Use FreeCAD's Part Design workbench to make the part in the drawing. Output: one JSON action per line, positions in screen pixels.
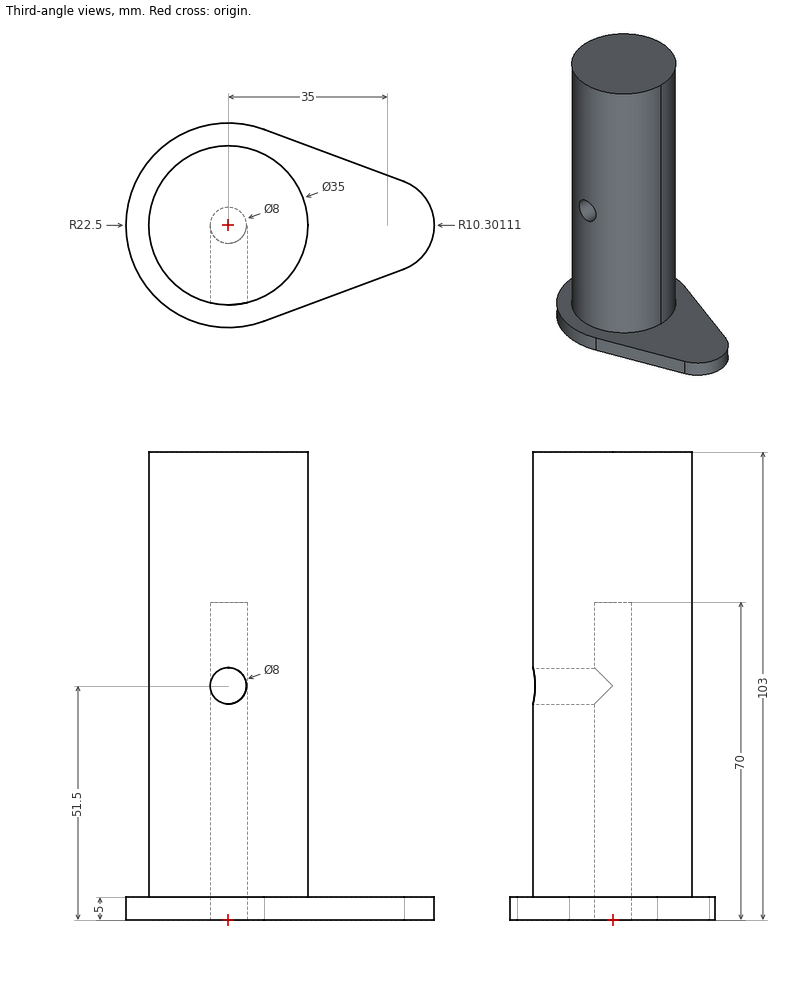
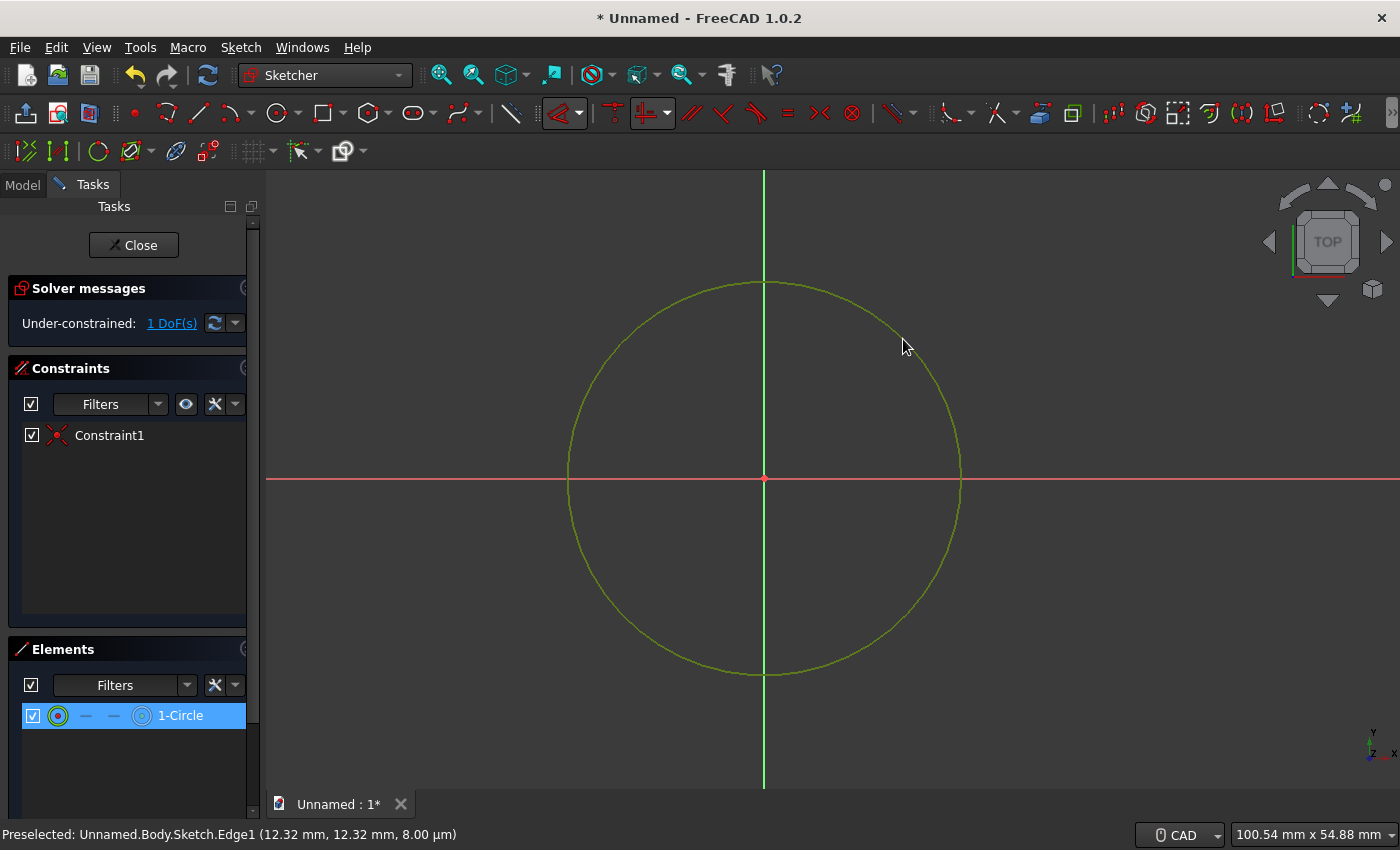
{"action": "key", "text": "k o"}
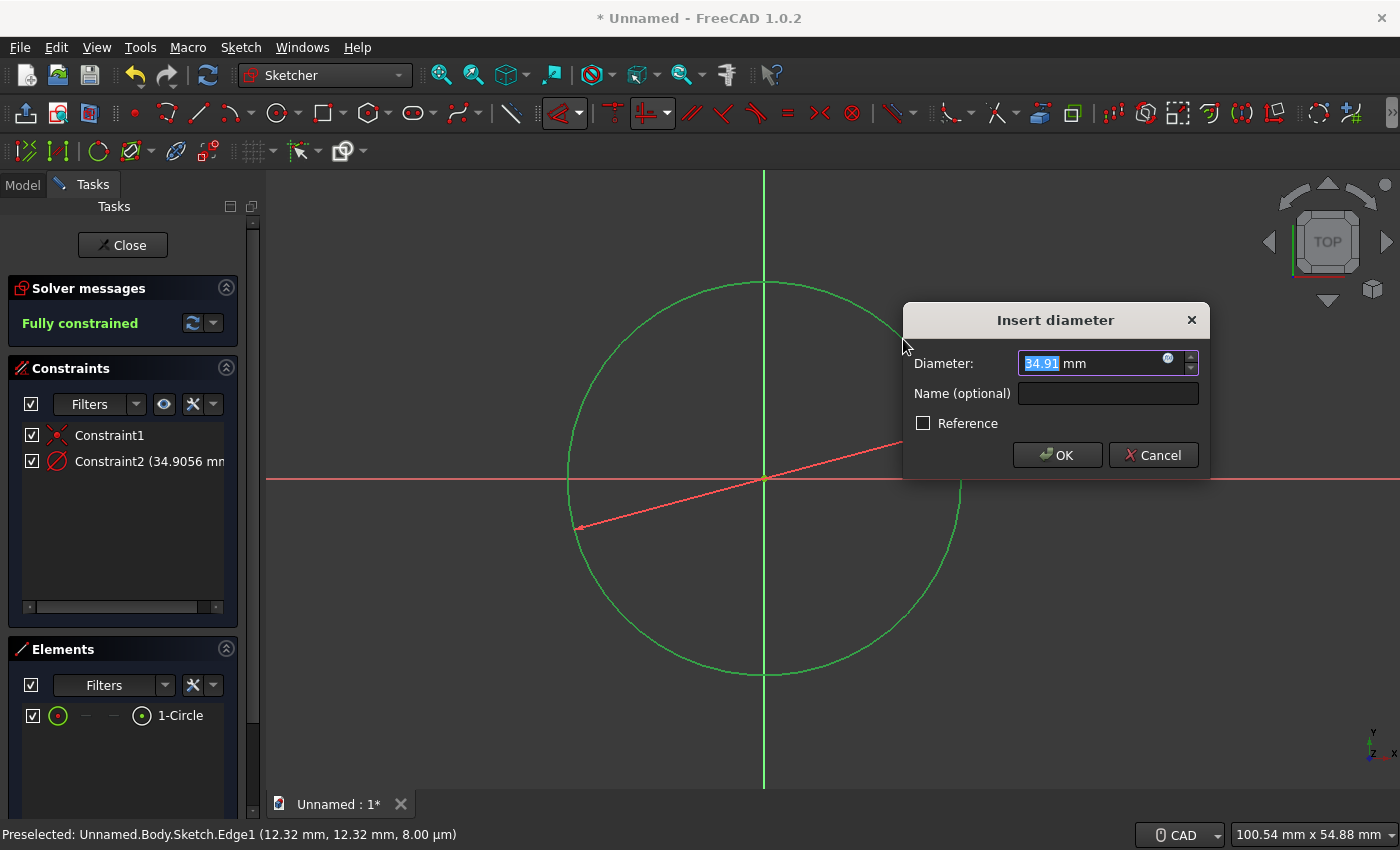
{"action": "type", "text": "35"}
{"action": "key", "text": "Return"}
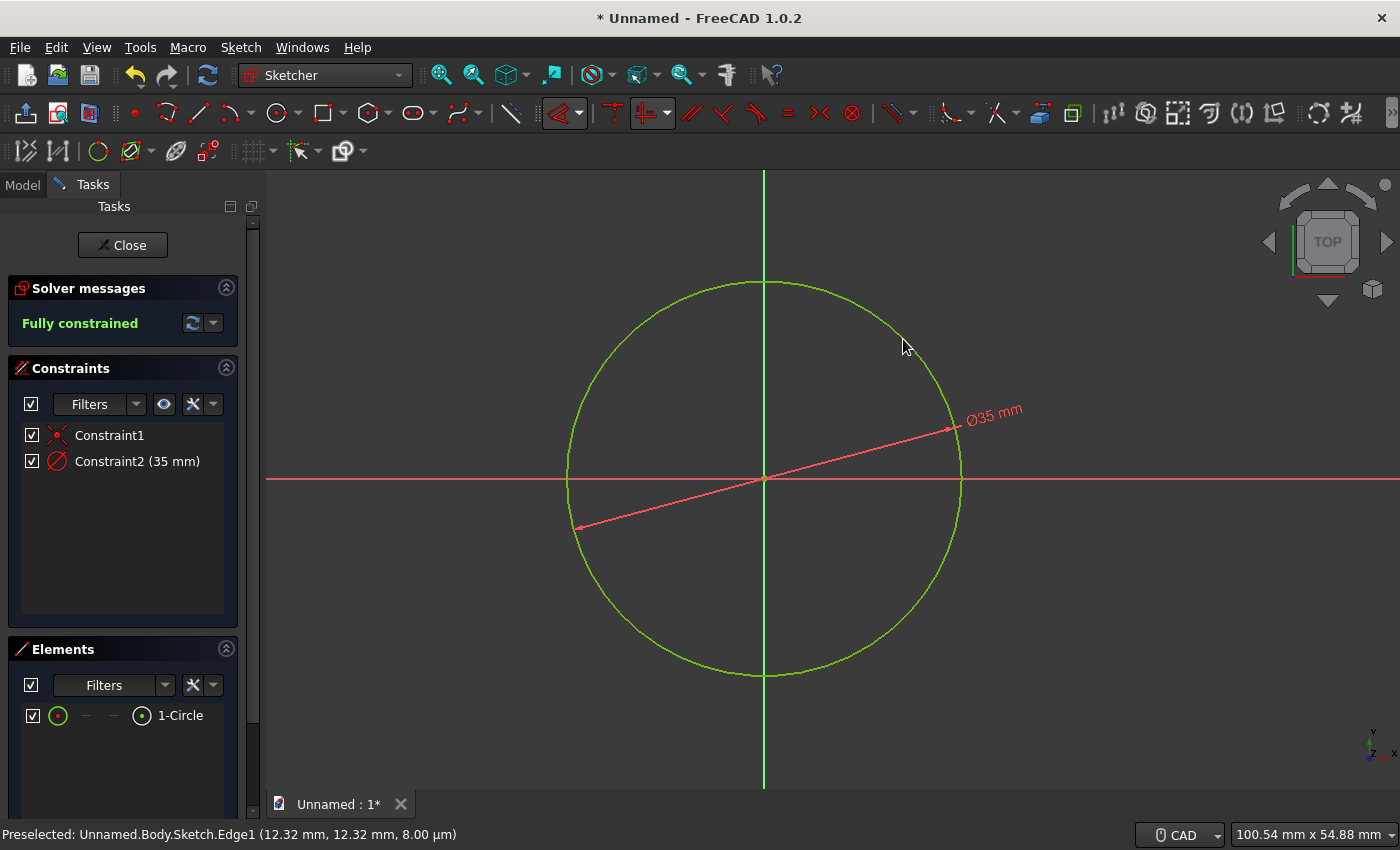
{"action": "left_click", "coordinate": [123, 245]}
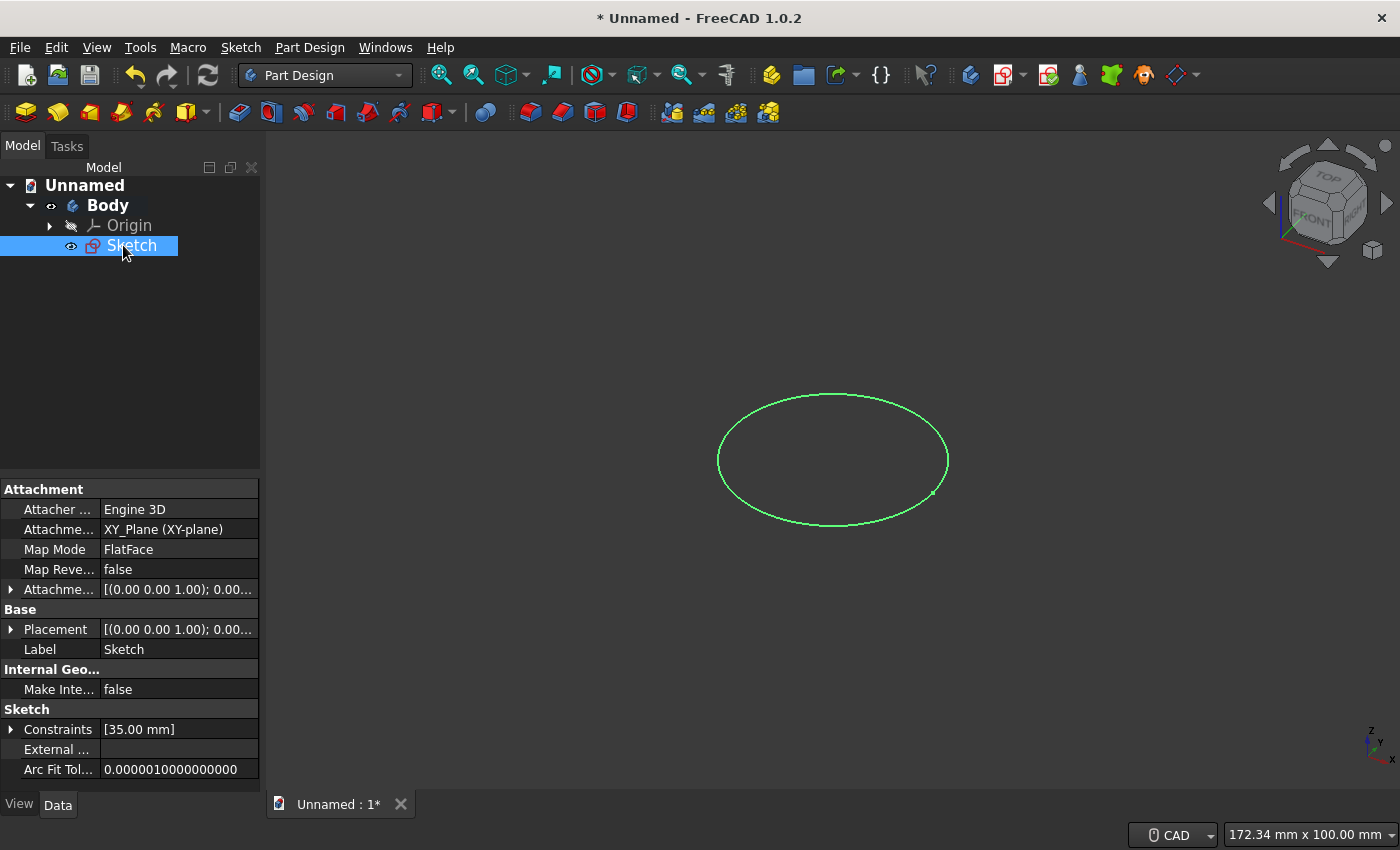
{"action": "left_click", "coordinate": [26, 112]}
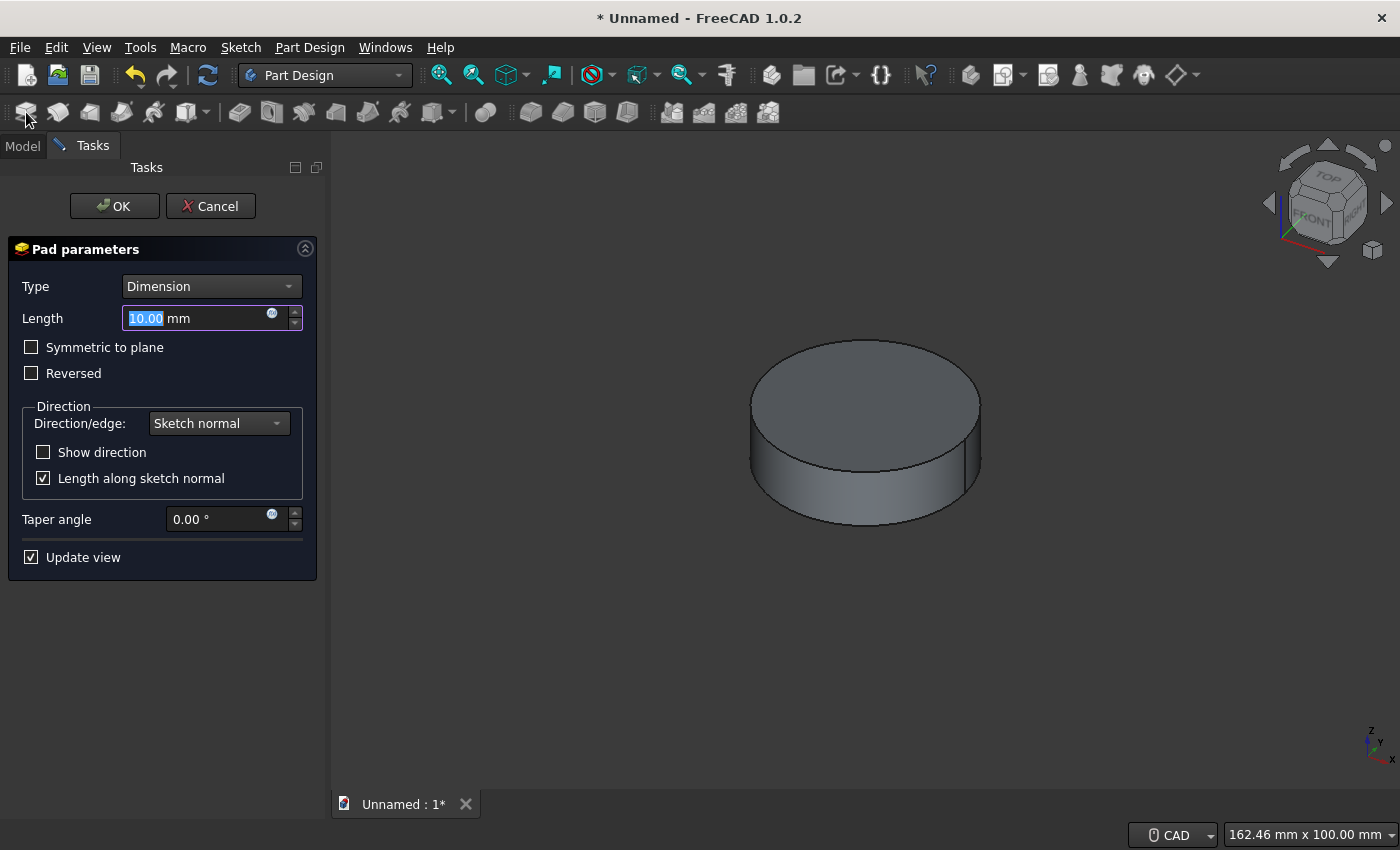
{"action": "type", "text": "103"}
{"action": "key", "text": "Tab"}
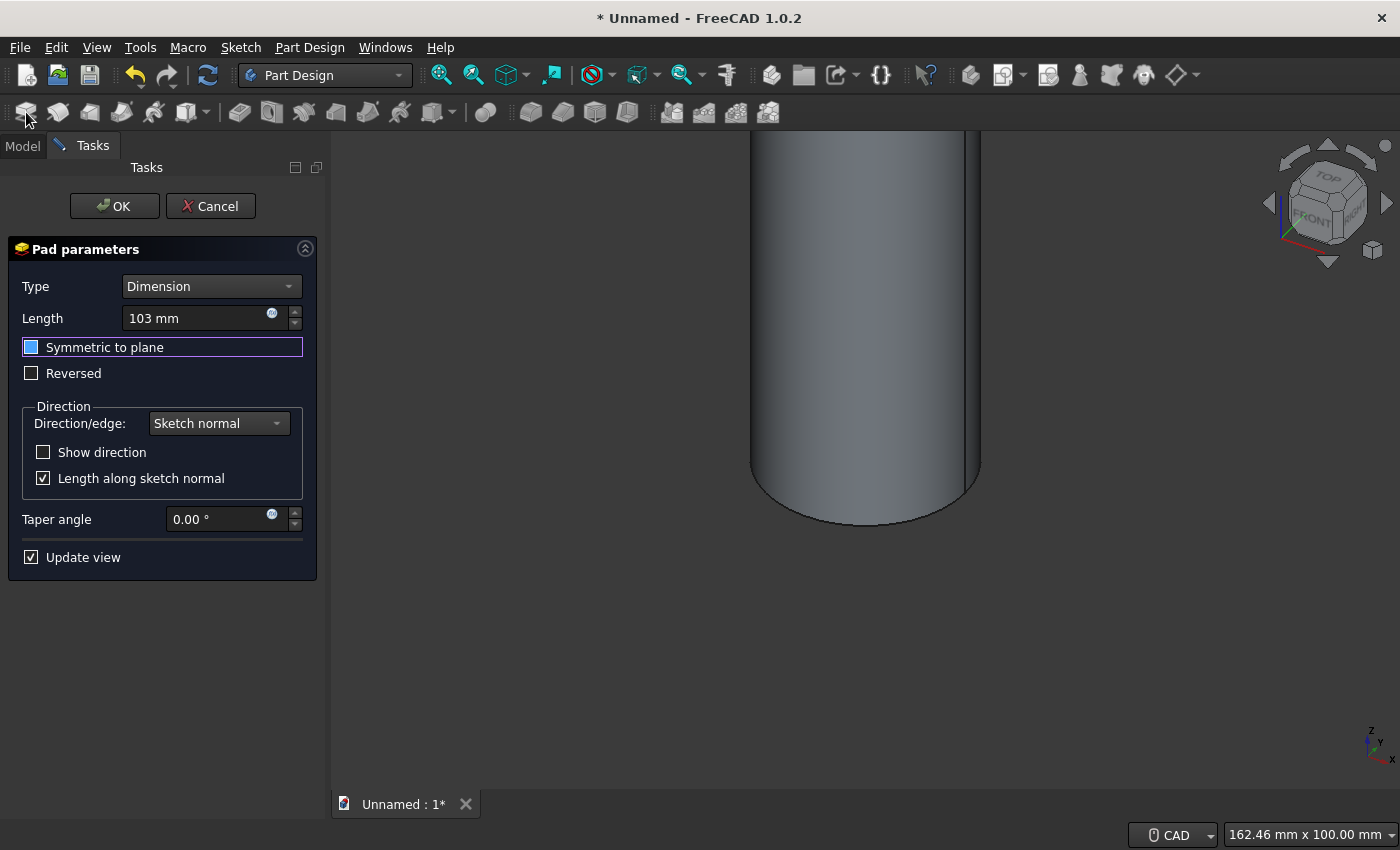
{"action": "left_click", "coordinate": [115, 206]}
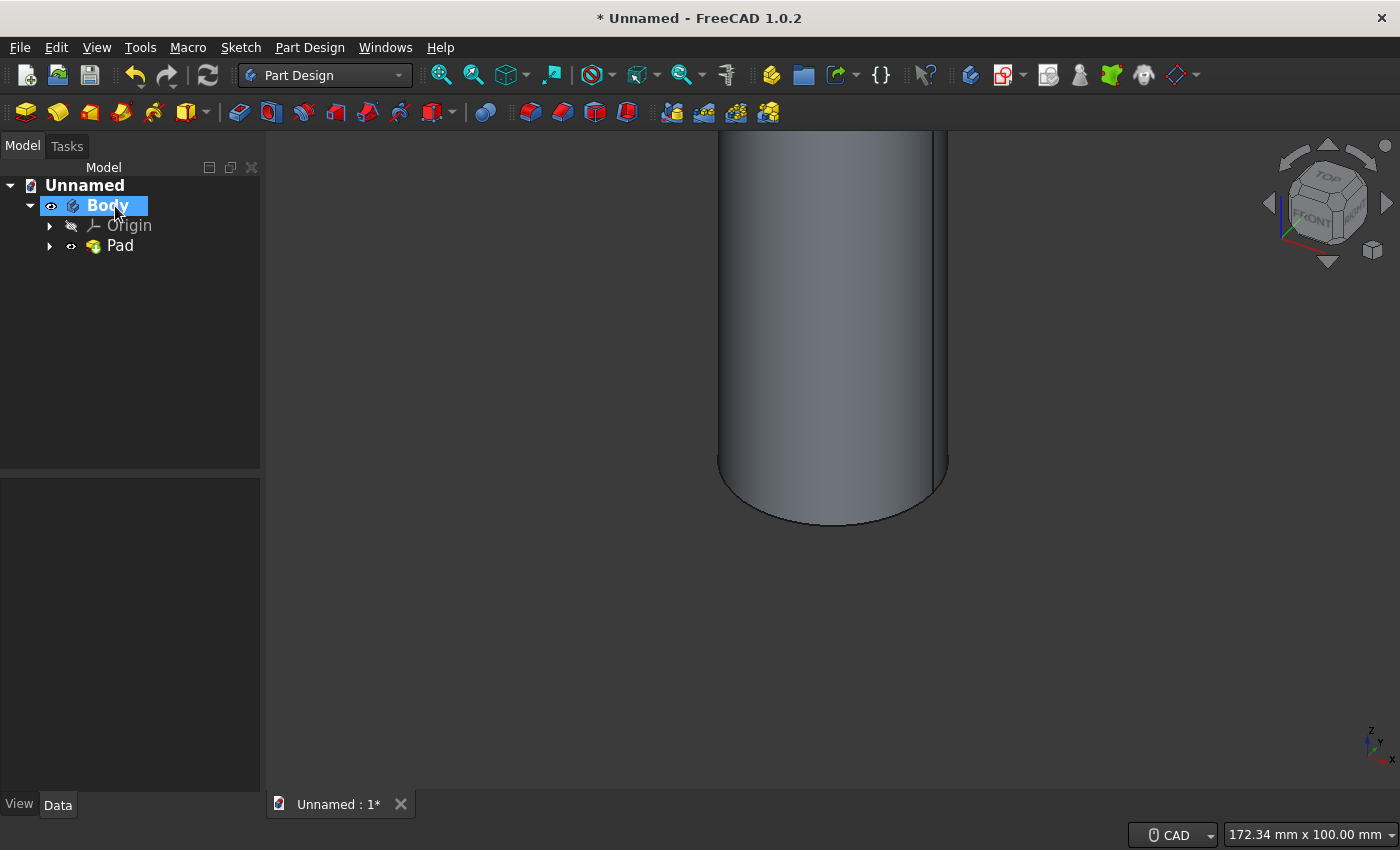
{"action": "left_click", "coordinate": [442, 76]}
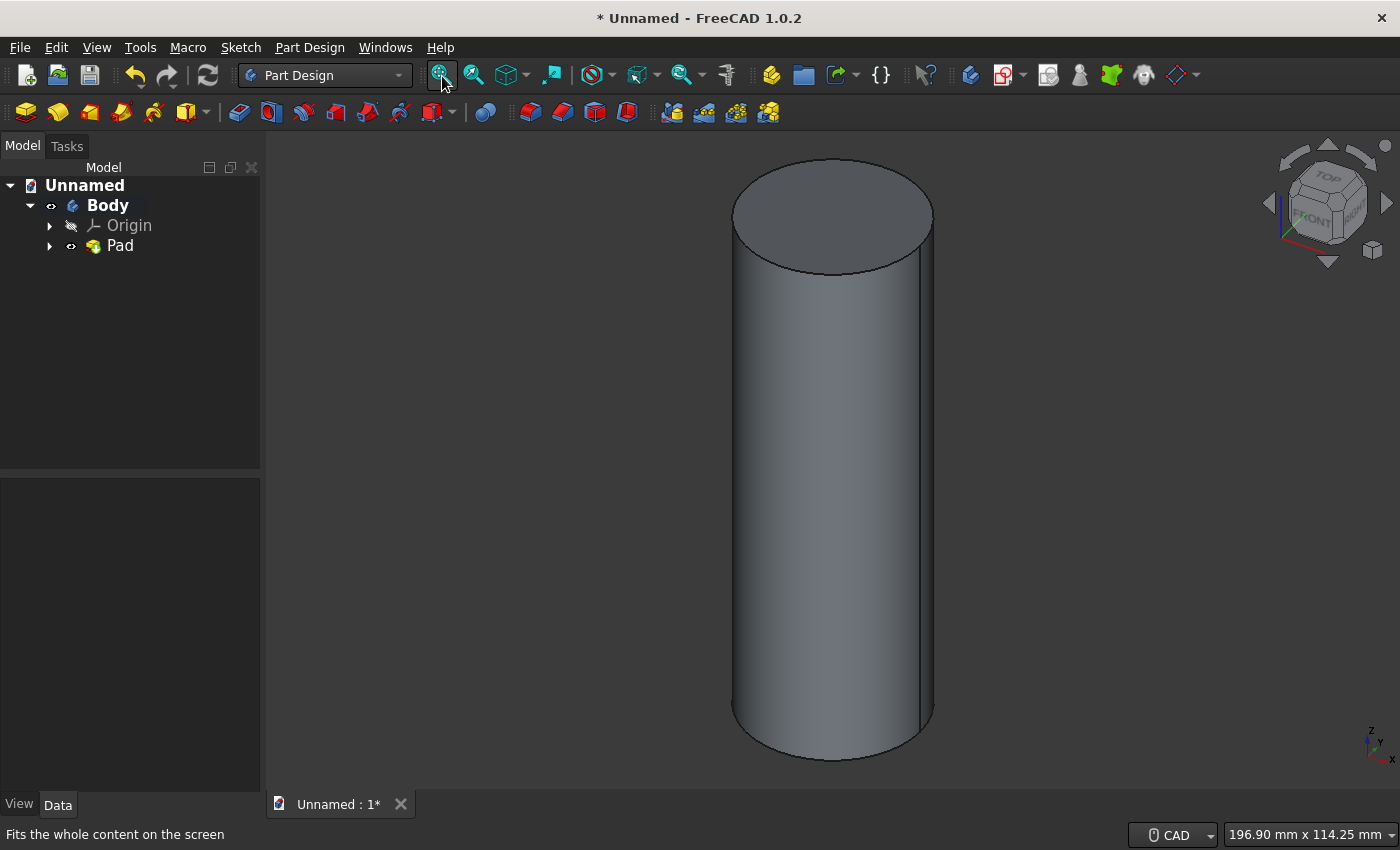
{"action": "left_click", "coordinate": [1004, 76]}